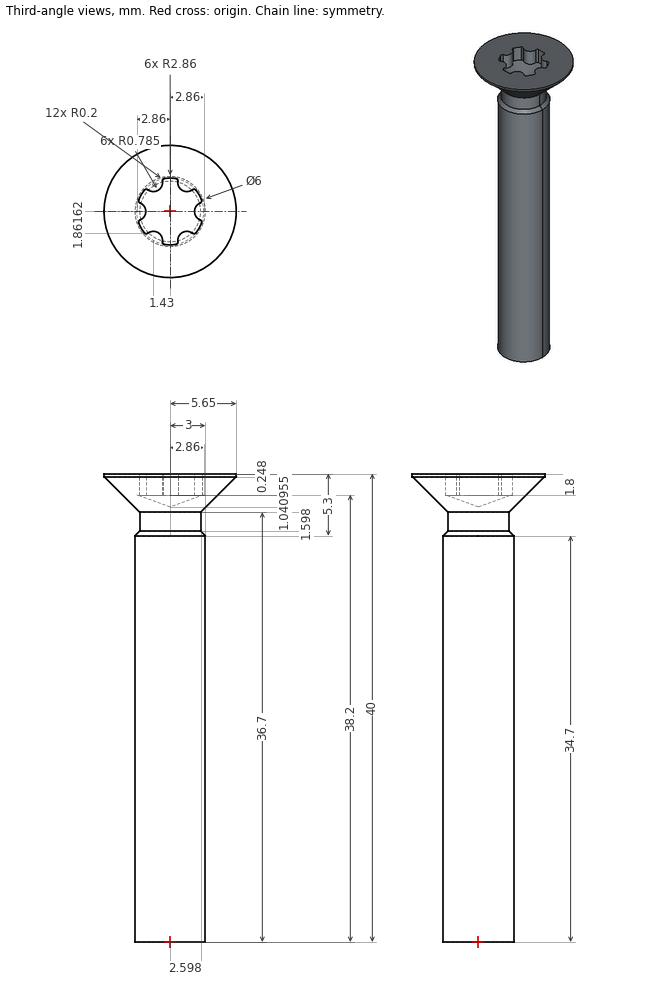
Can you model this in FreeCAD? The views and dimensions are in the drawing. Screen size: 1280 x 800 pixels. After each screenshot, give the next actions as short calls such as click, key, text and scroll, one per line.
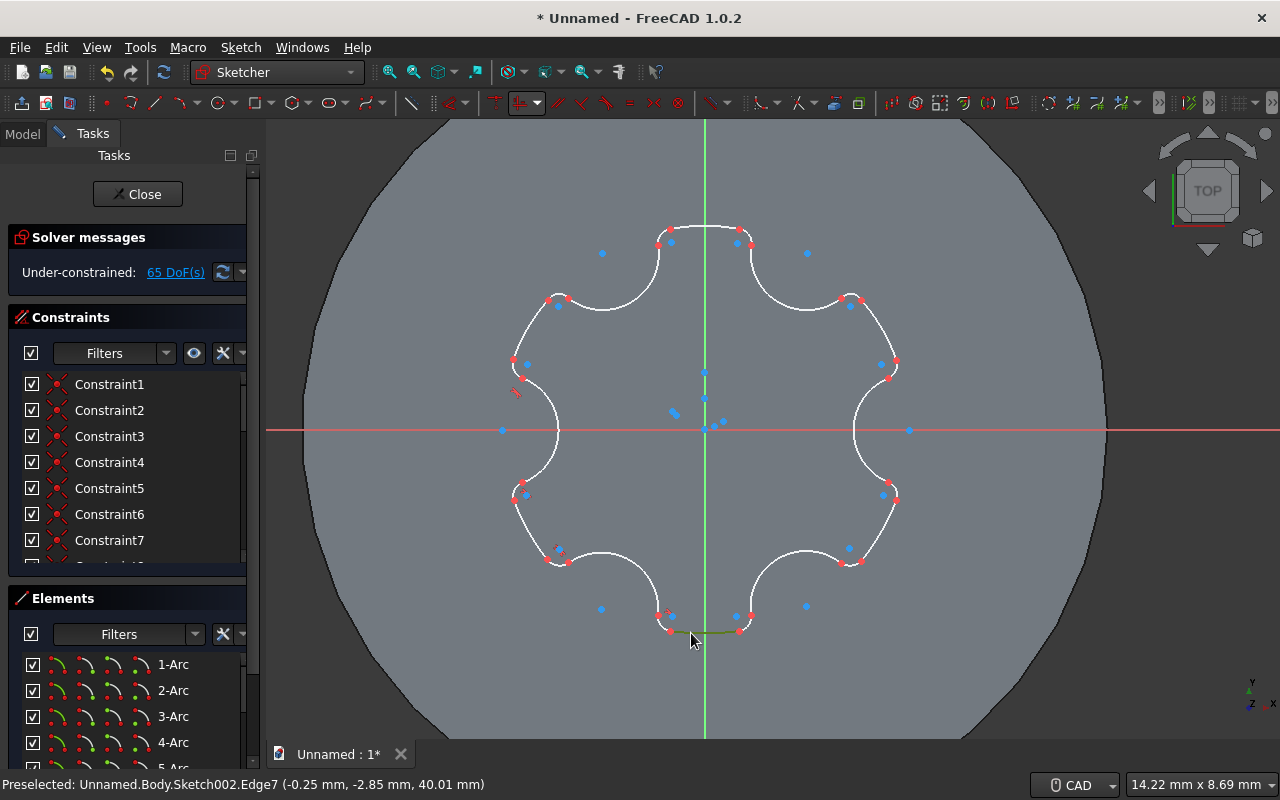
scroll(748, 625, up, 2)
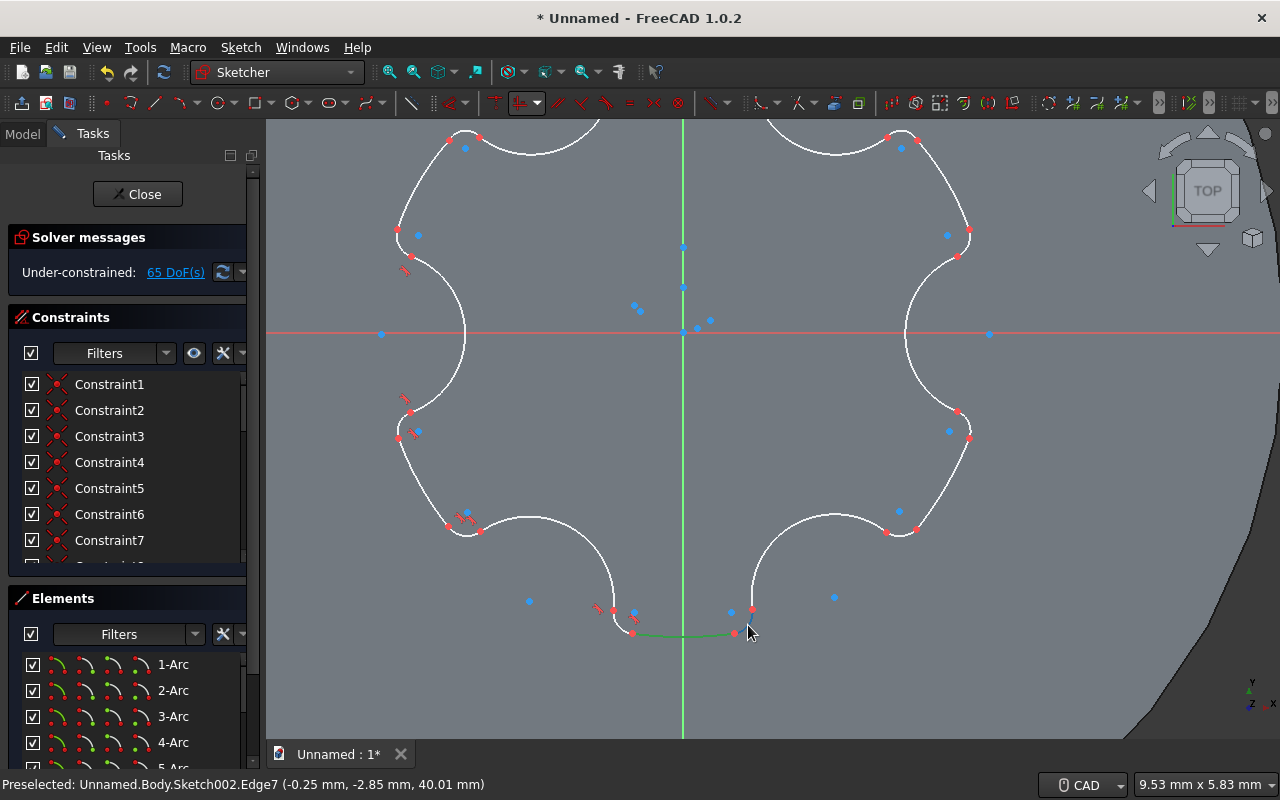
click(748, 625)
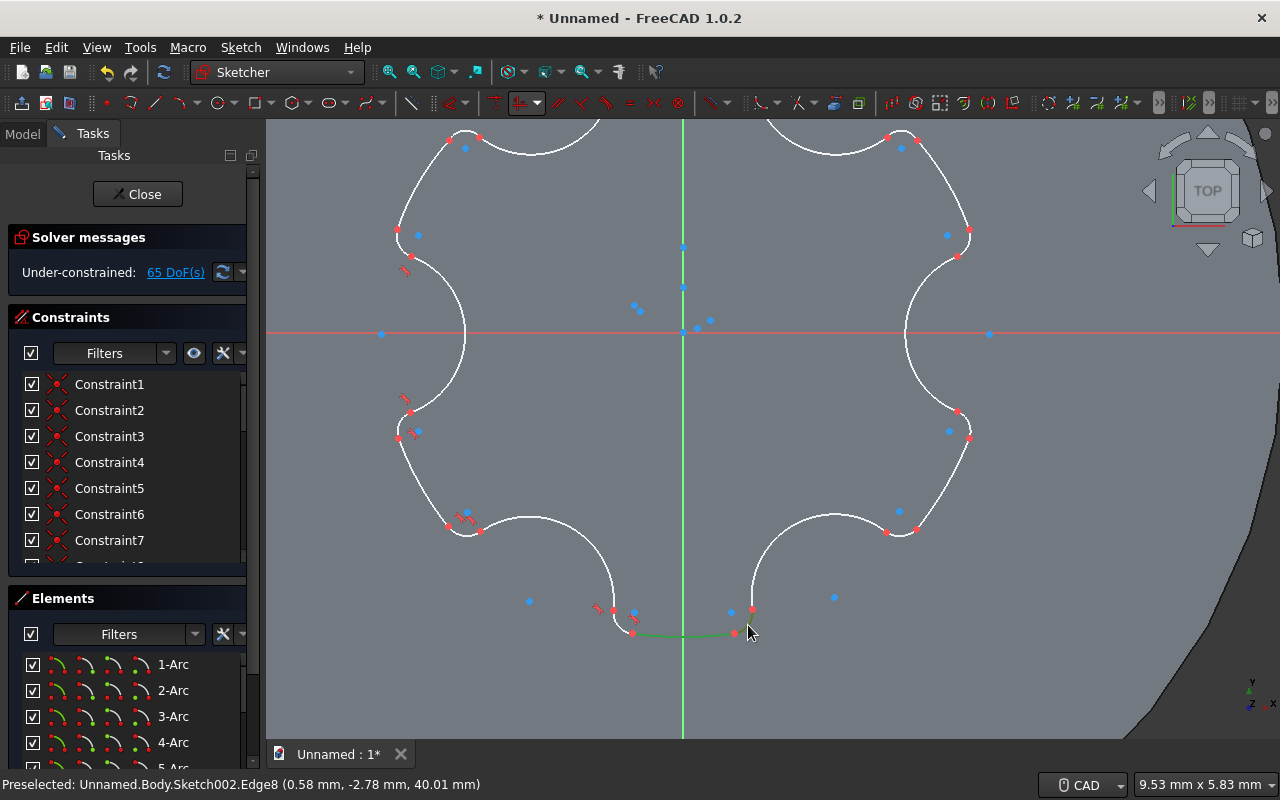
click(606, 104)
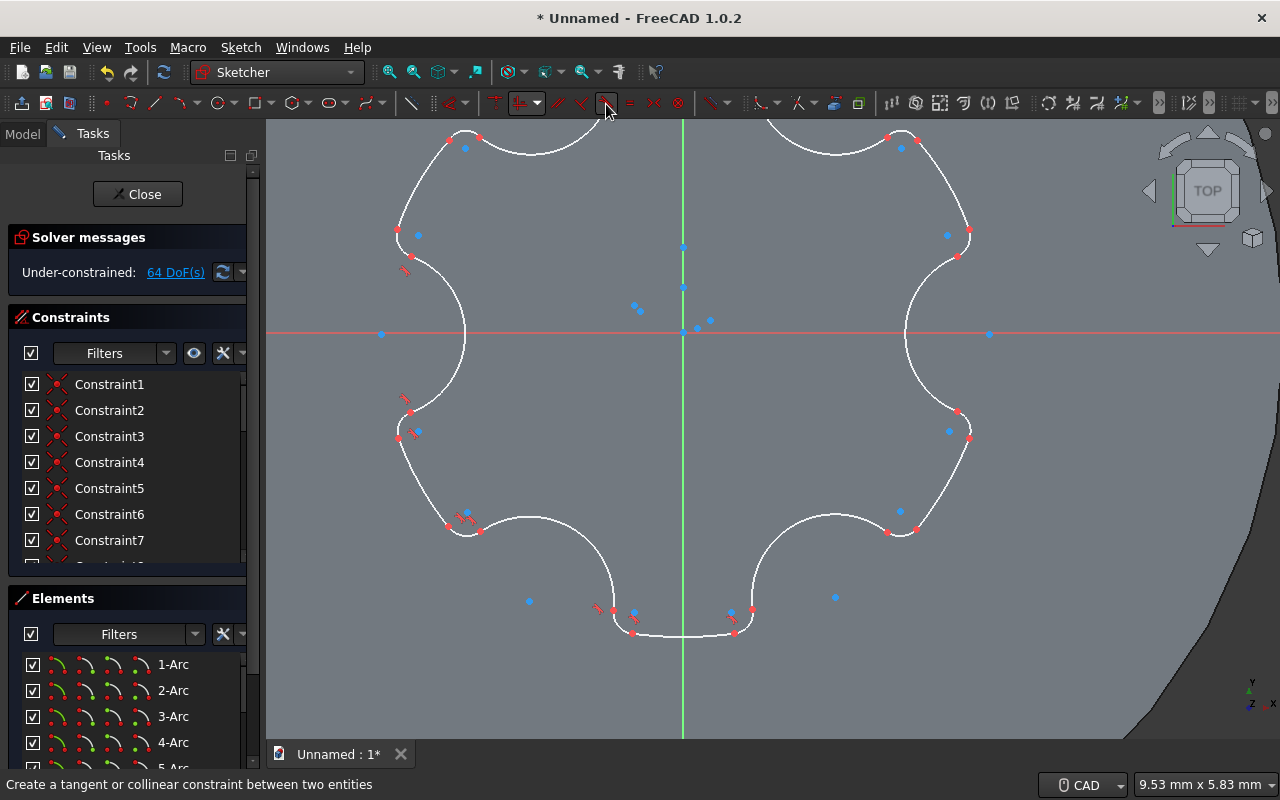
scroll(744, 630, up, 2)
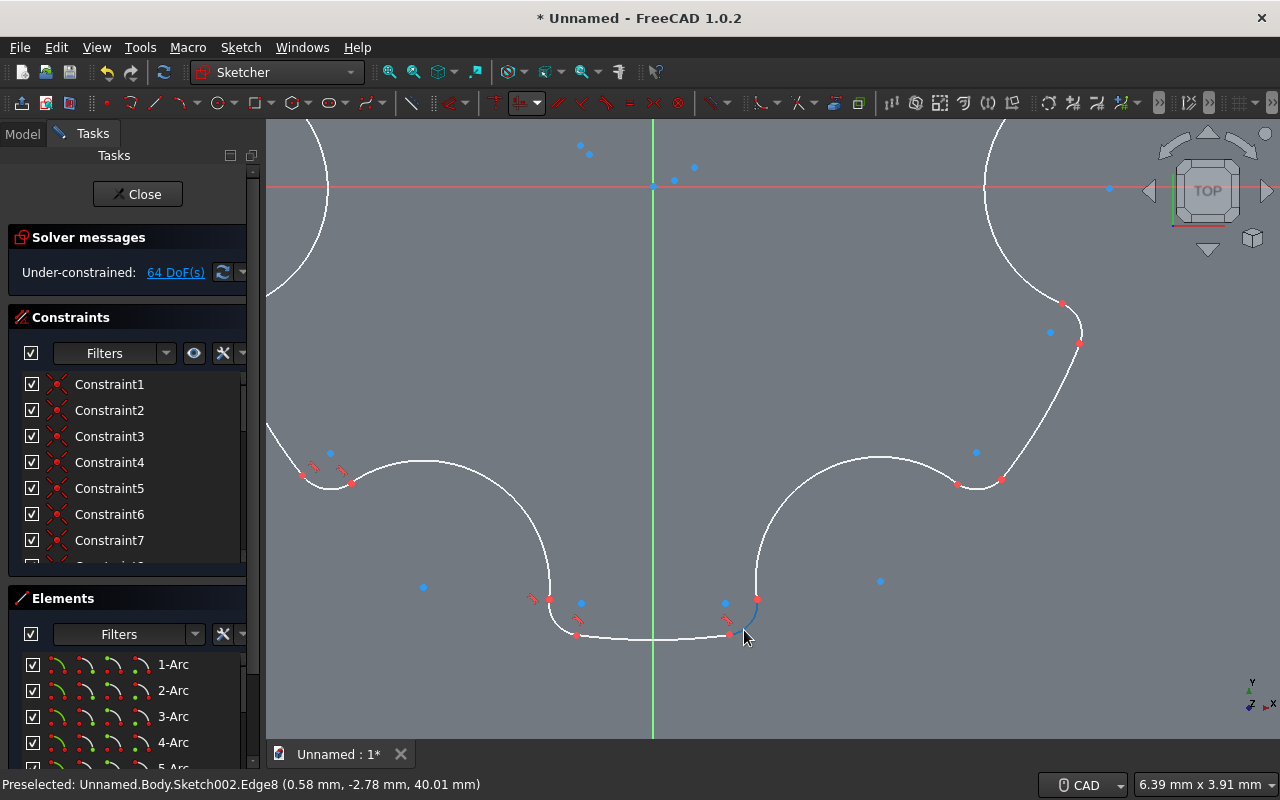
click(744, 630)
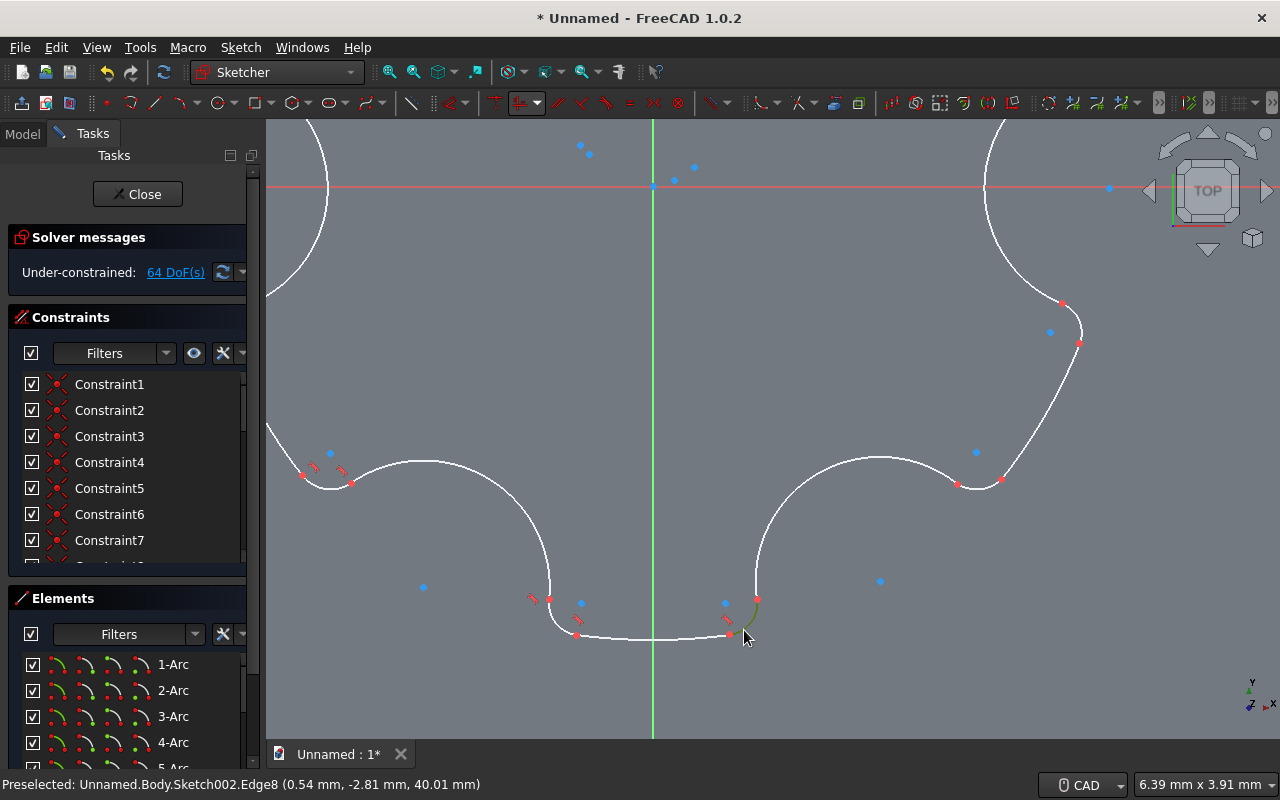
click(875, 457)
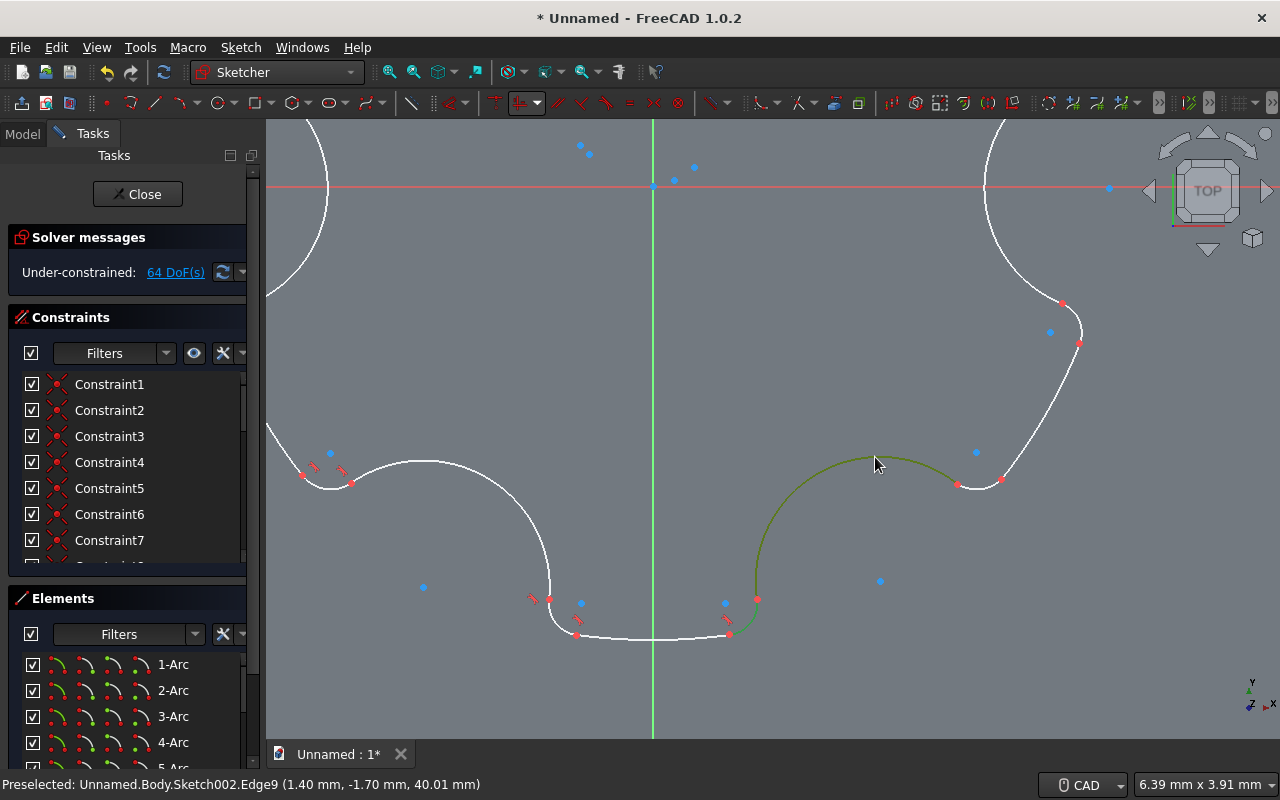
click(606, 104)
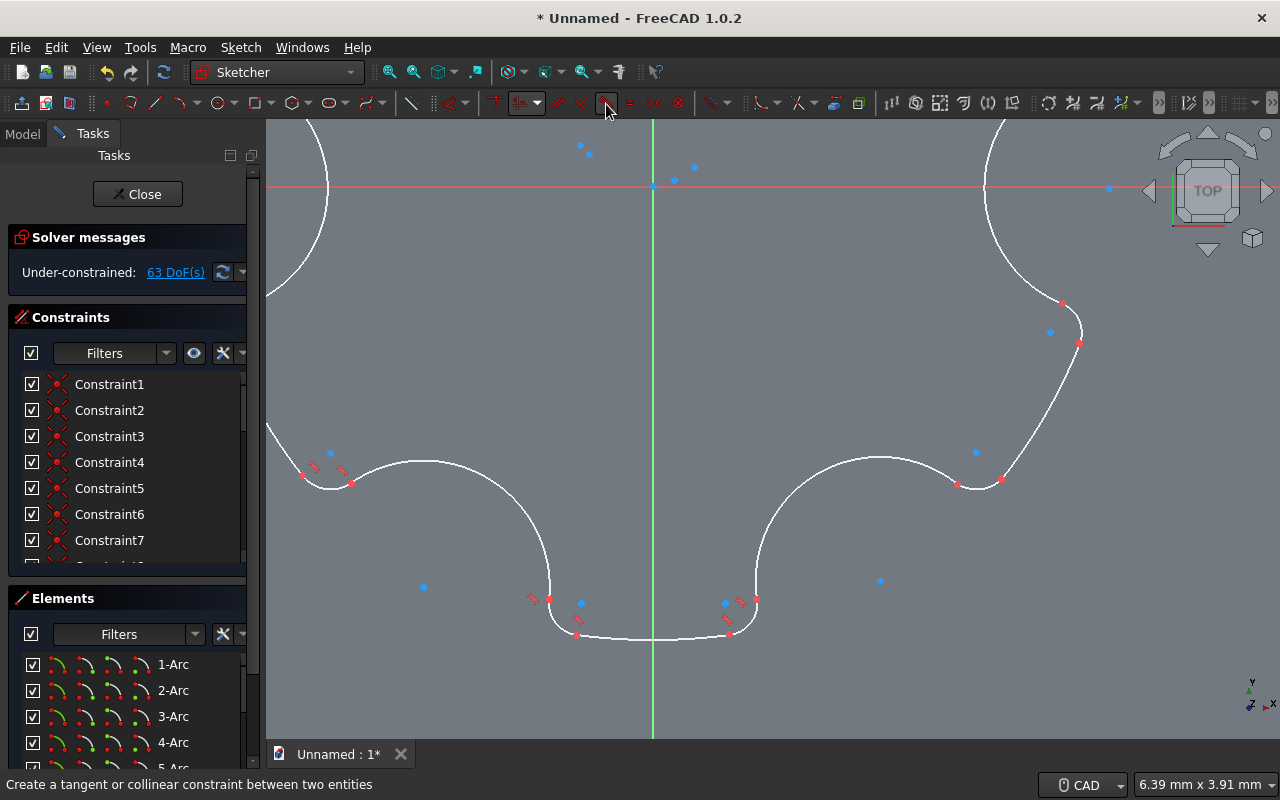
click(875, 457)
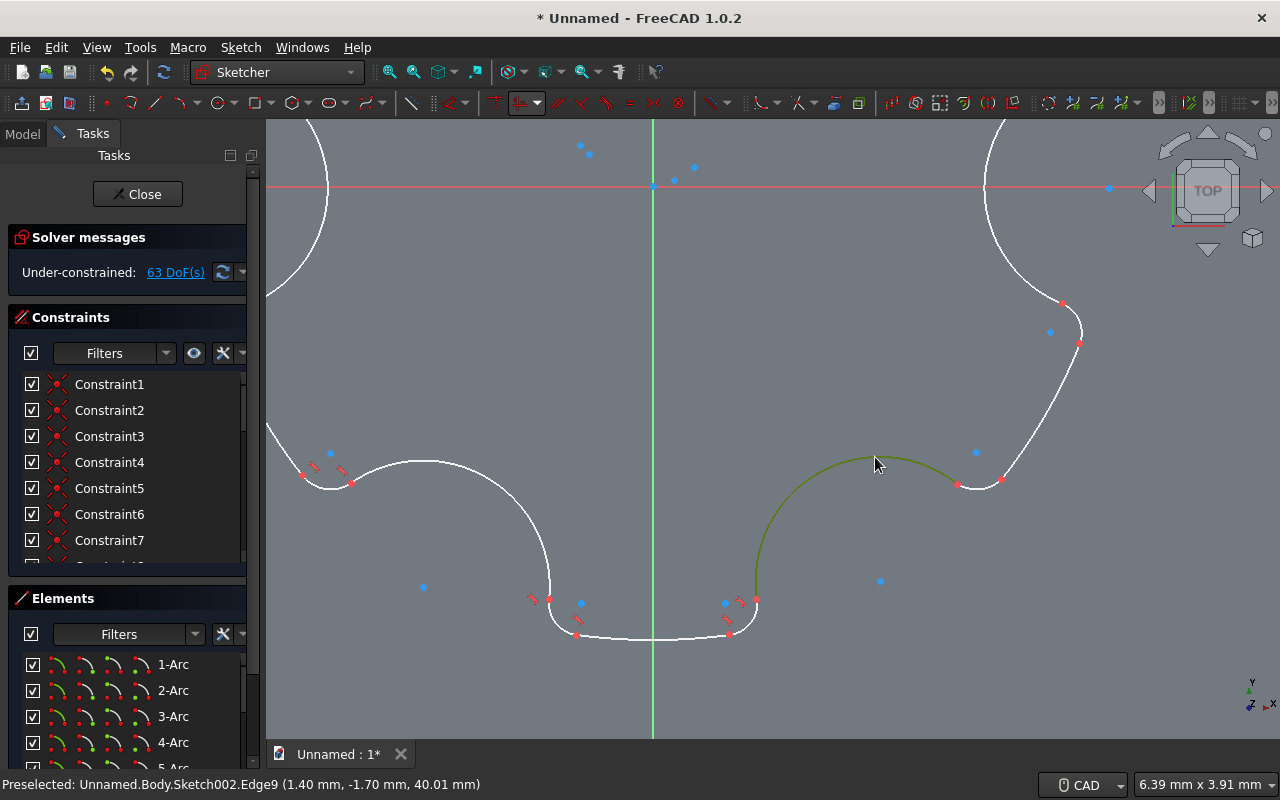
click(971, 489)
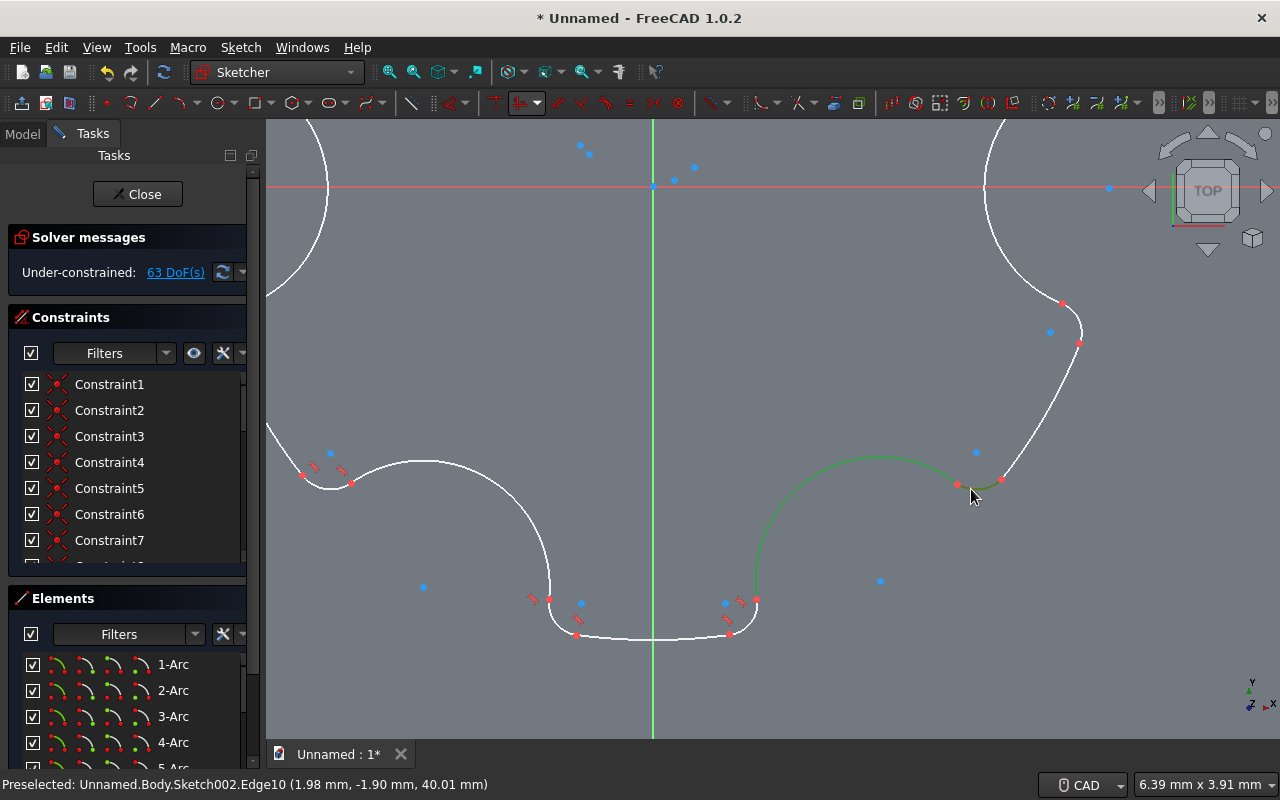
key(t)